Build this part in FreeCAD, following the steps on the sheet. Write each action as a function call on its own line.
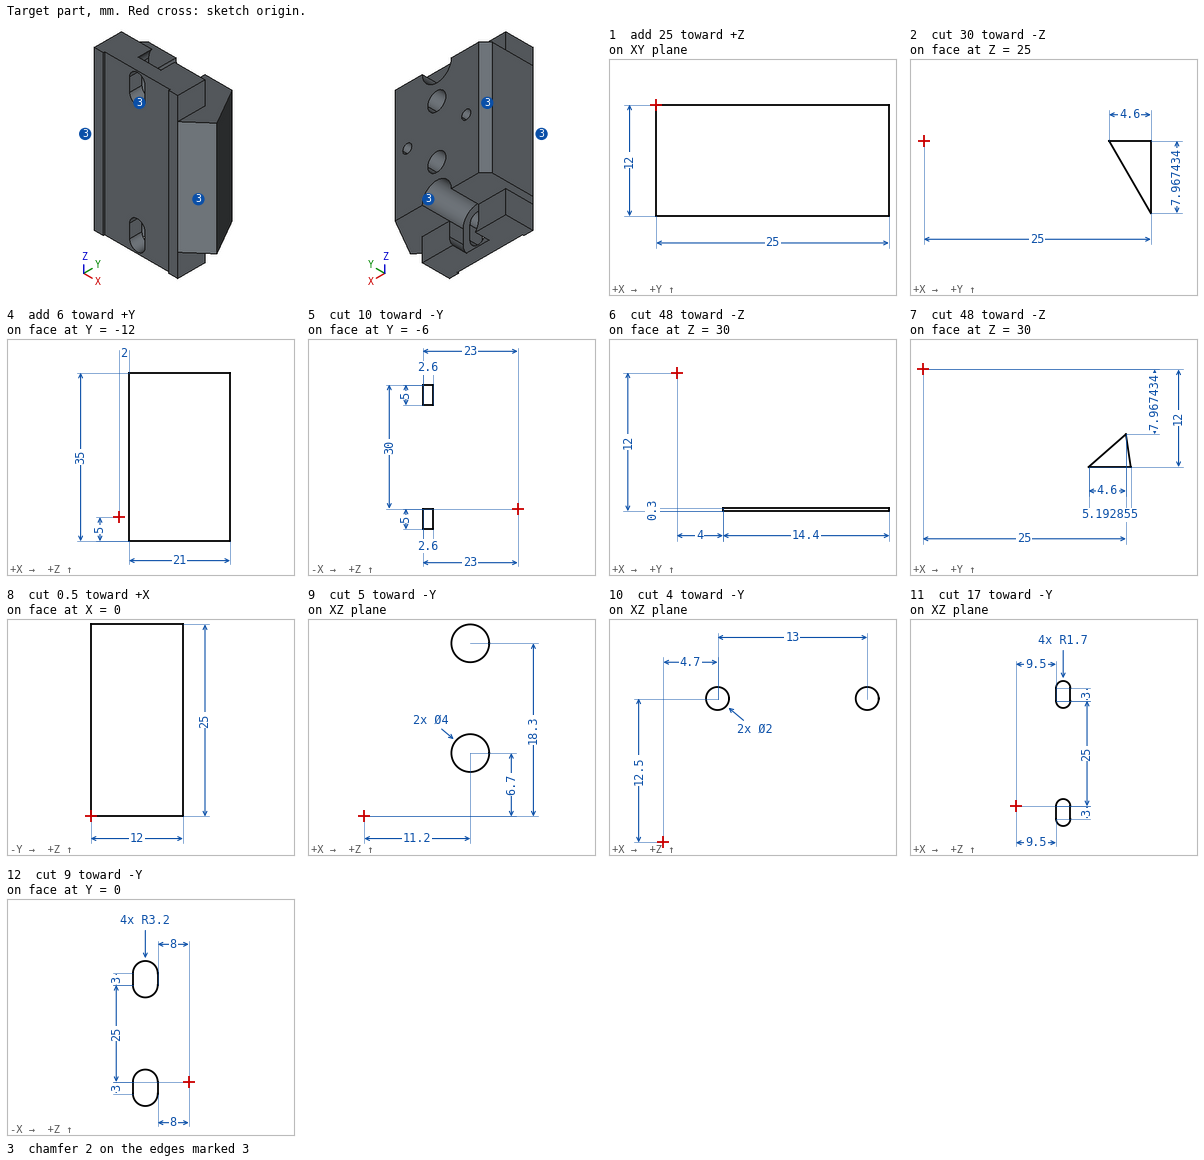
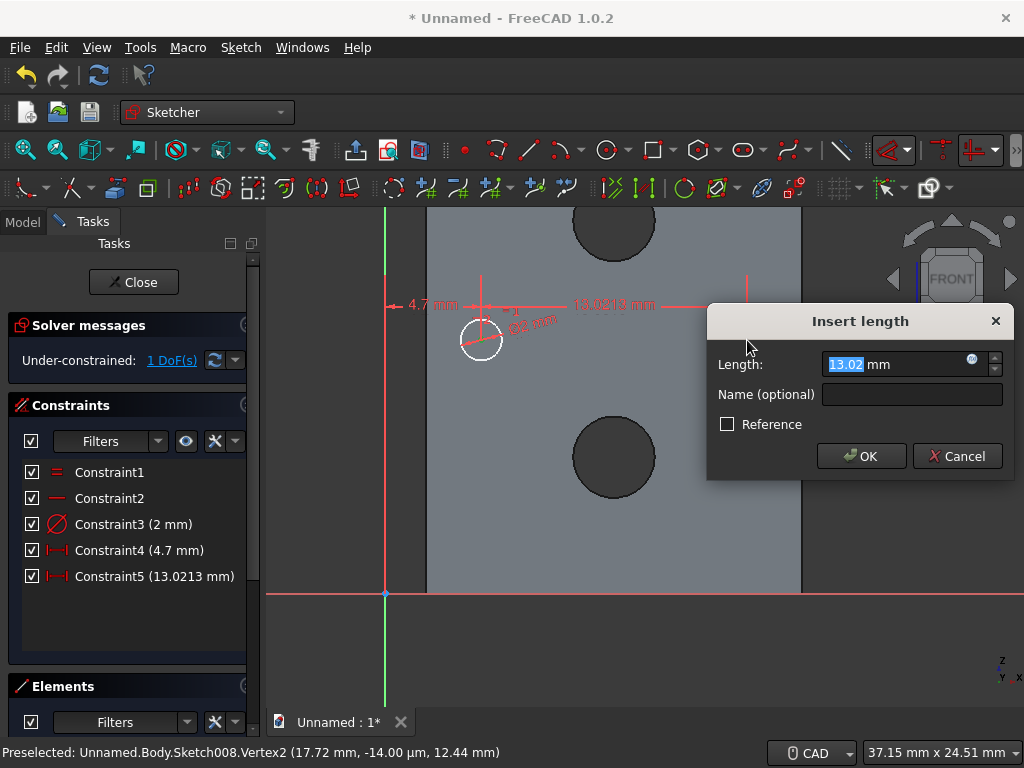
text(13)
key(Return)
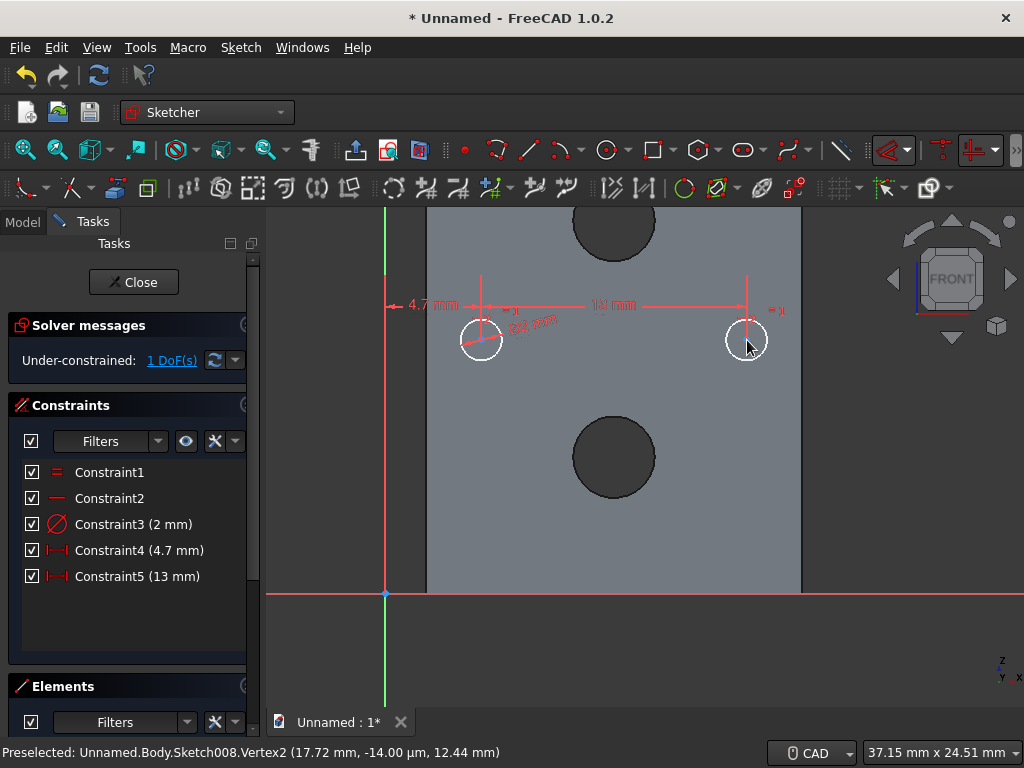
click(481, 340)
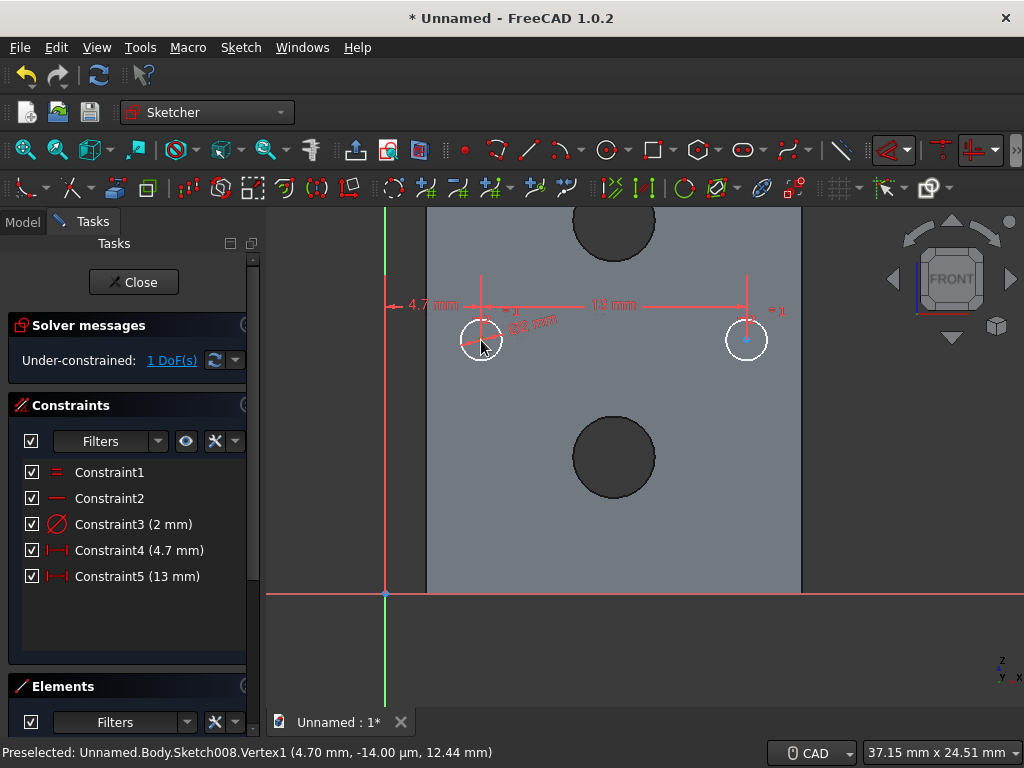
key(i)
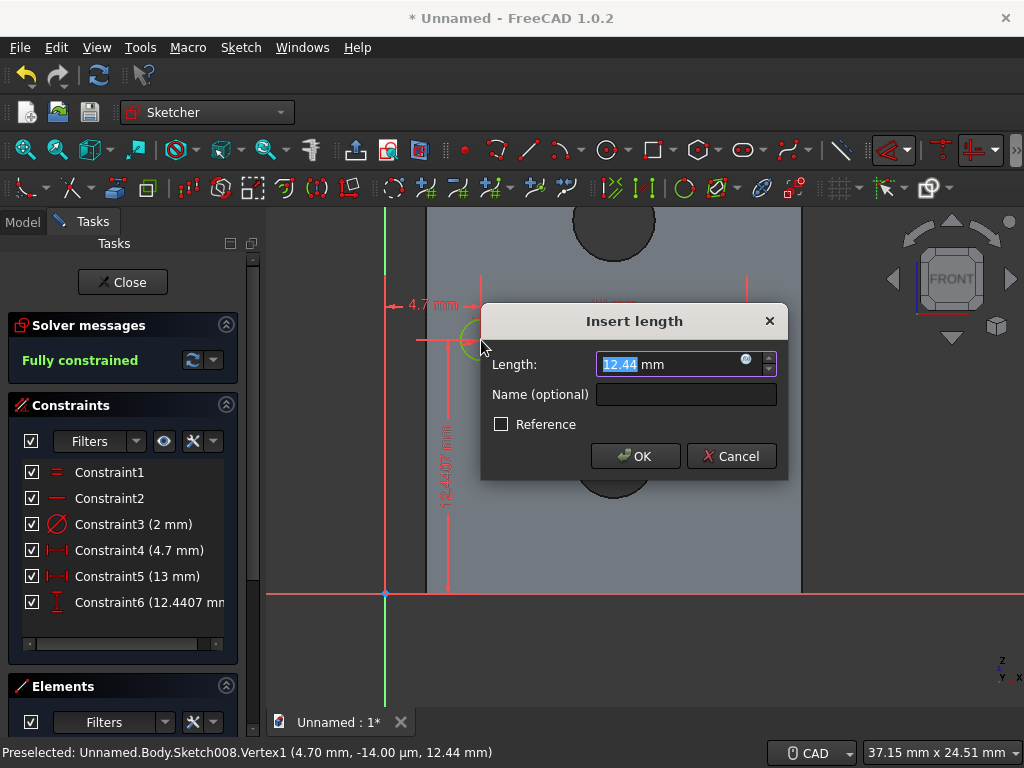
text(12.5)
key(Return)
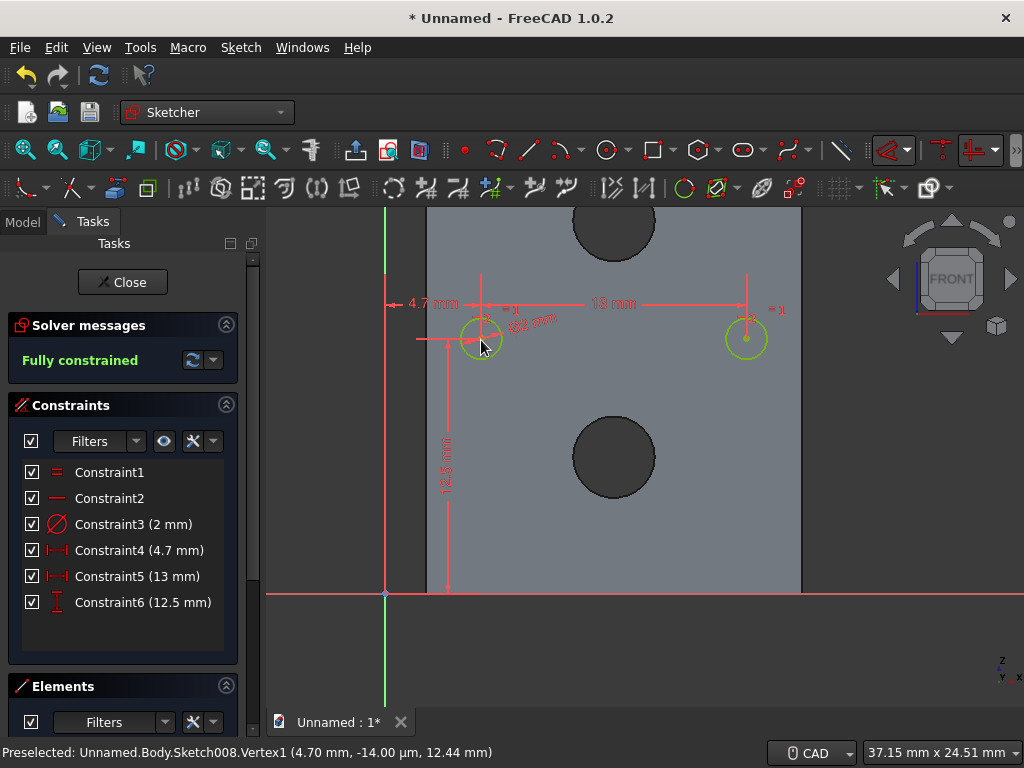
click(123, 282)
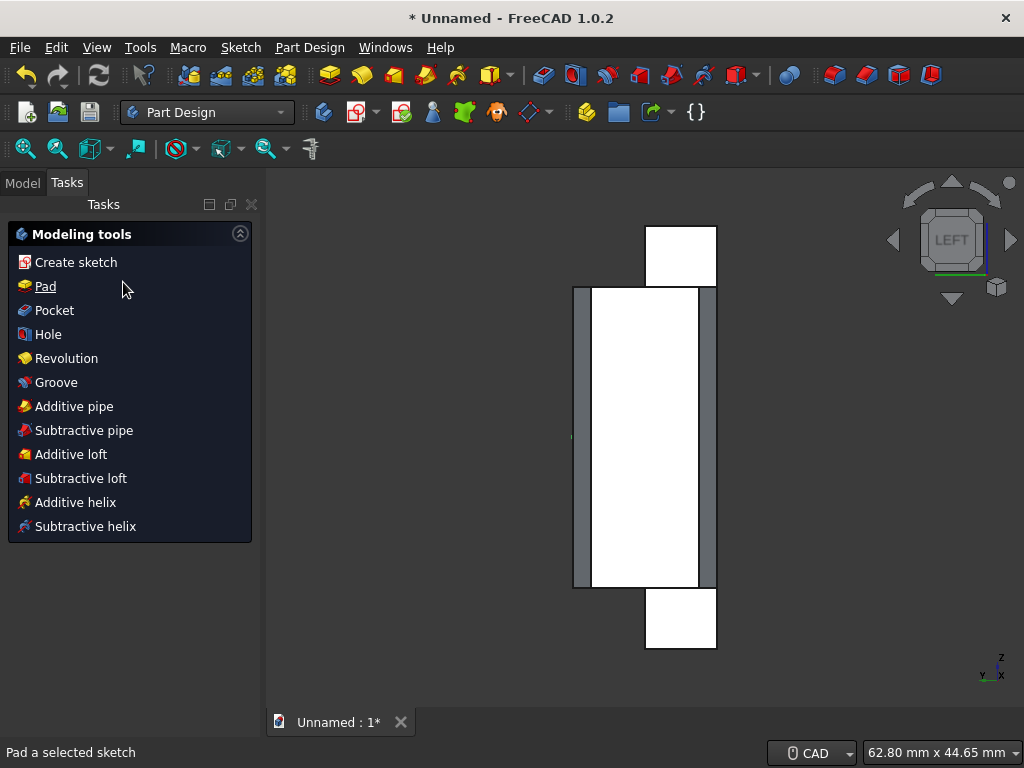
click(544, 76)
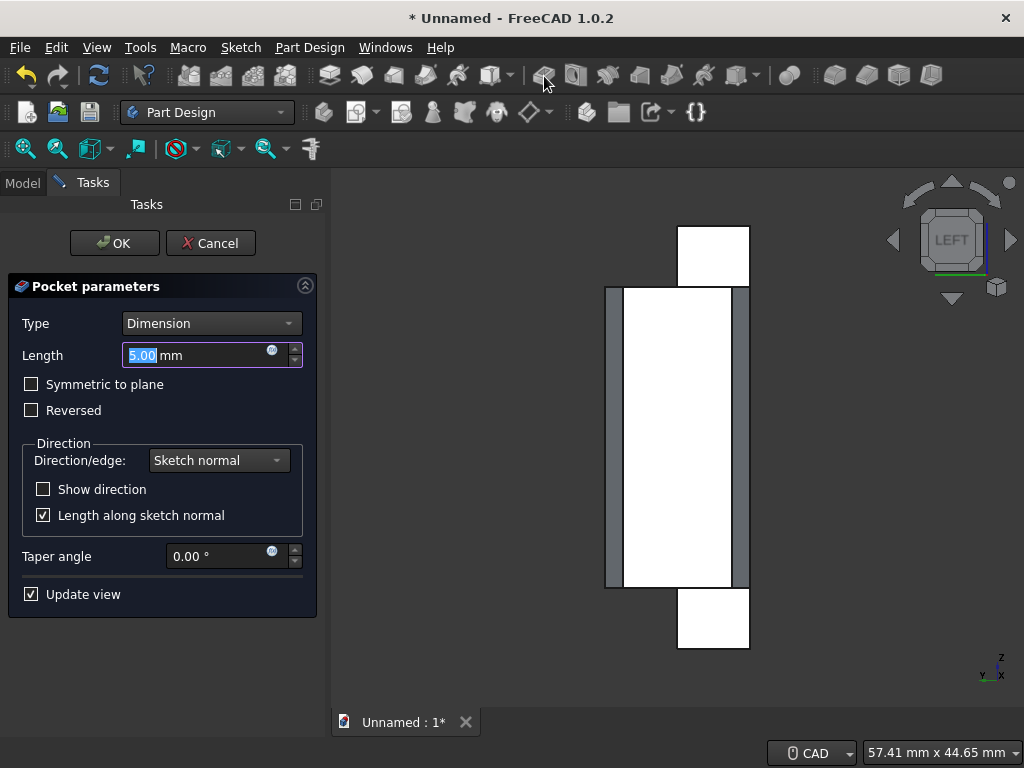
text(4)
key(Tab)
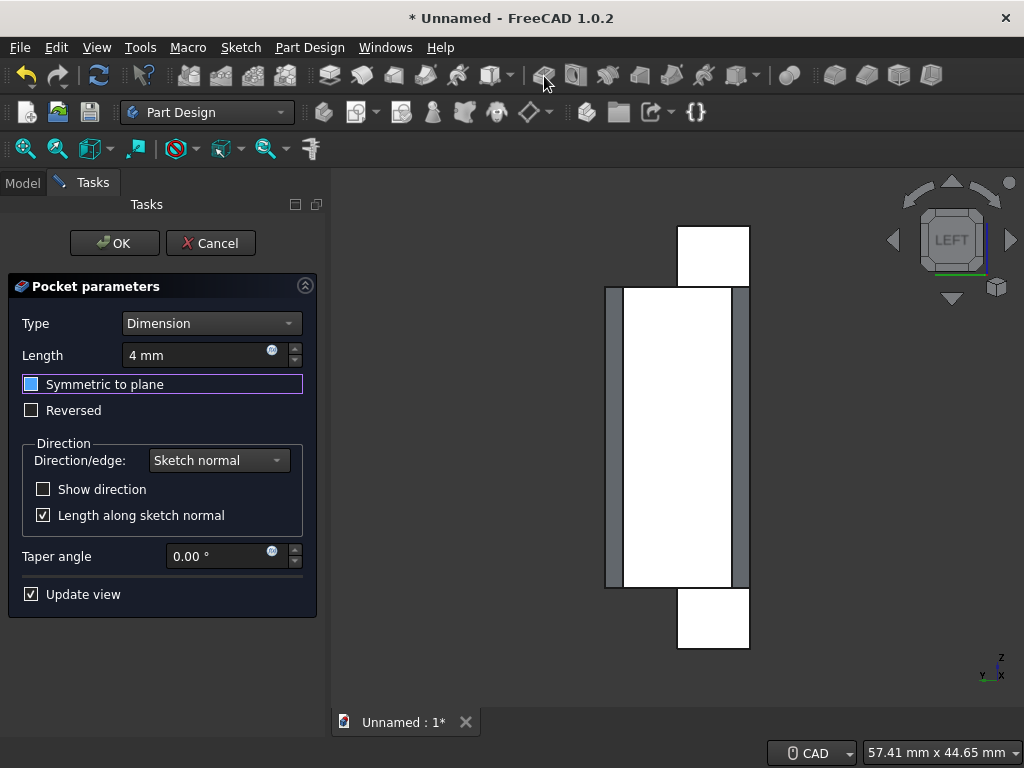
click(30, 410)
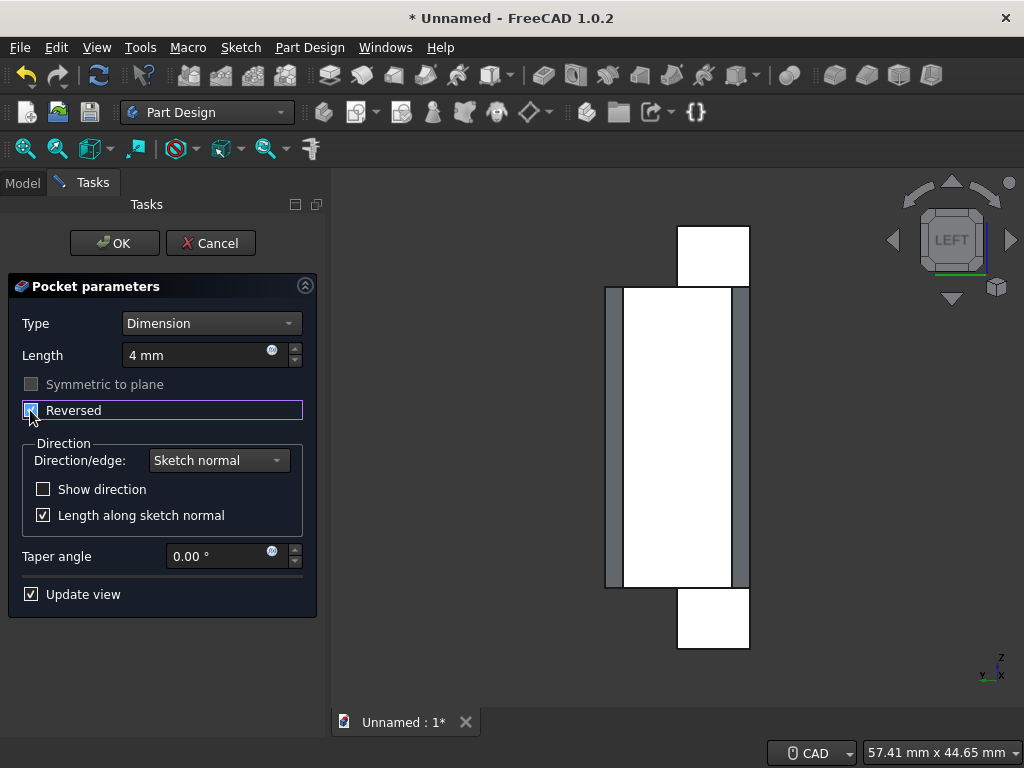
click(115, 243)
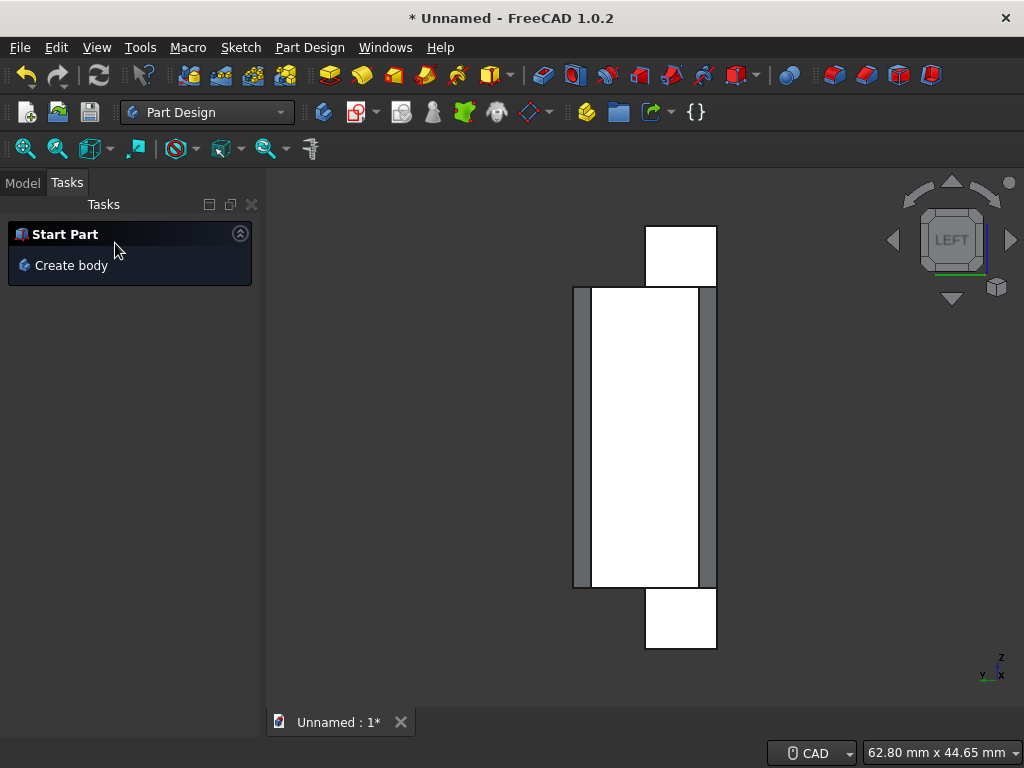
click(356, 112)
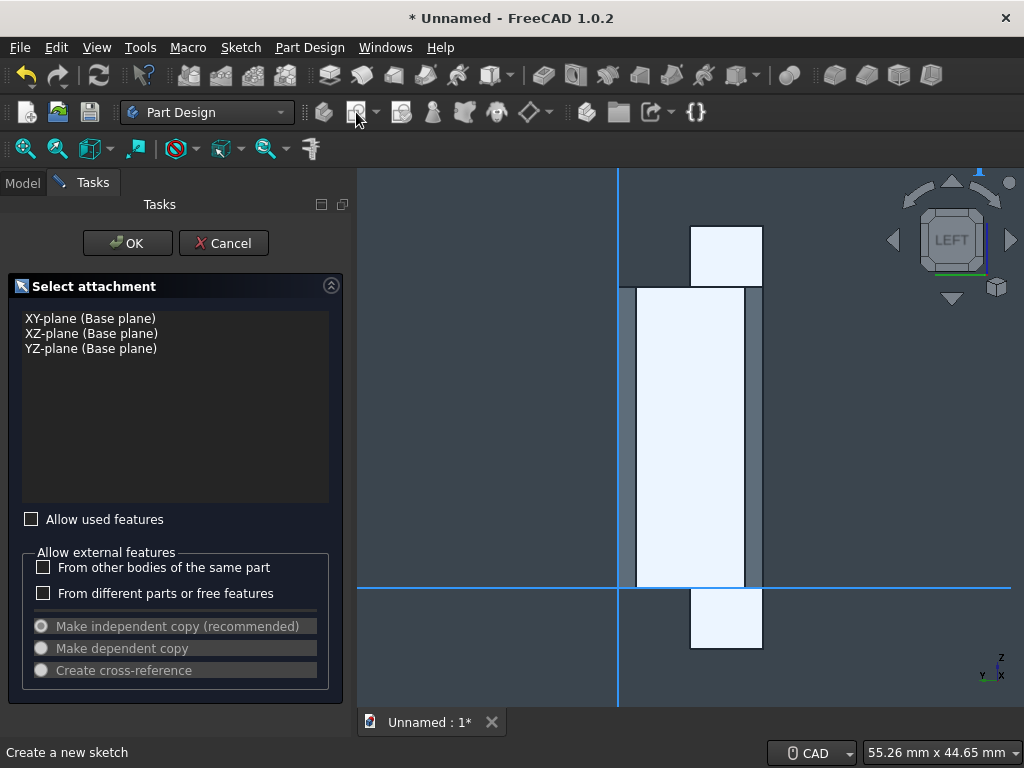
click(82, 334)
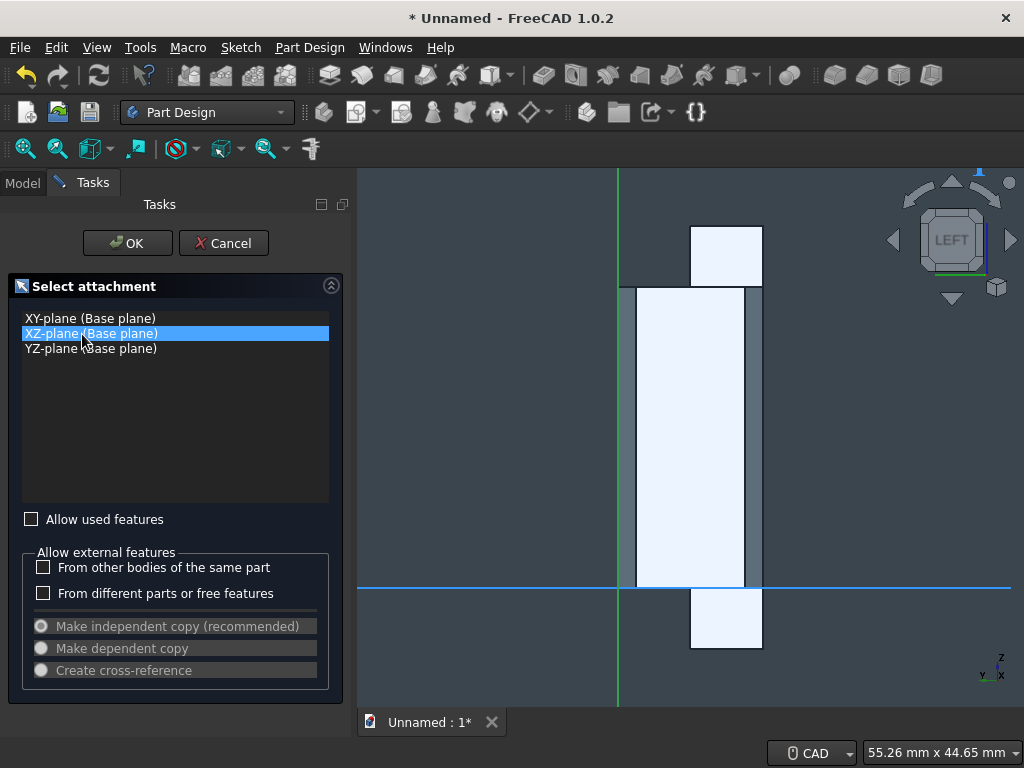
click(128, 243)